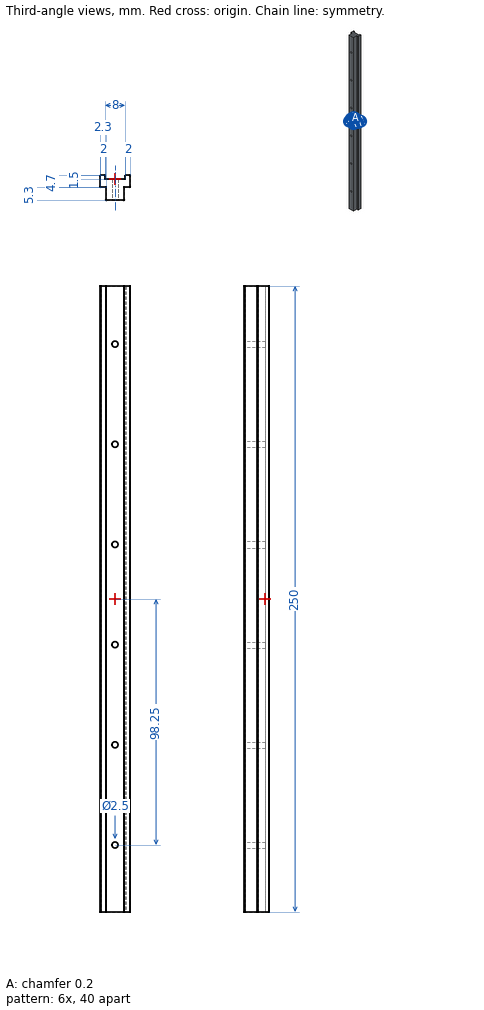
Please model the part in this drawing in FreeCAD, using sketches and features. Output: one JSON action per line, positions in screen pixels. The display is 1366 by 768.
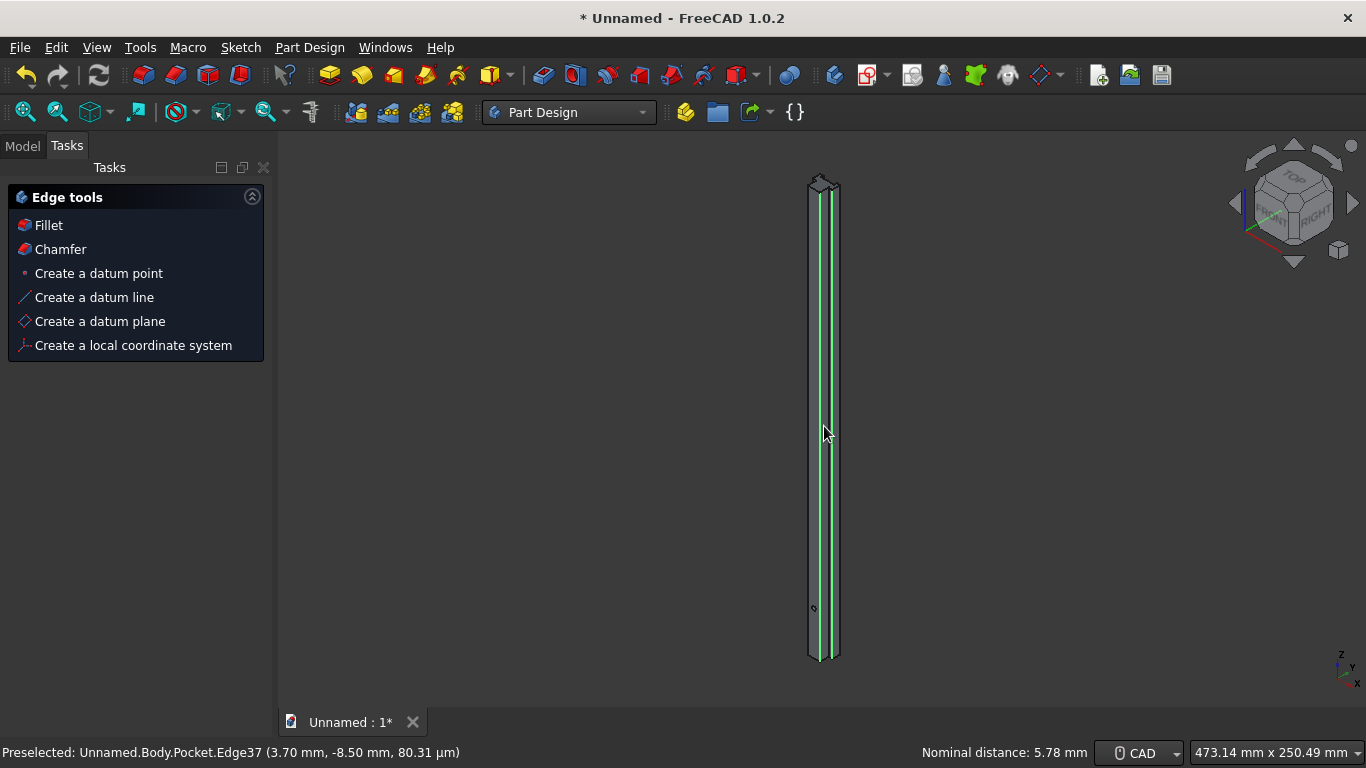
{"action": "key", "text": "2"}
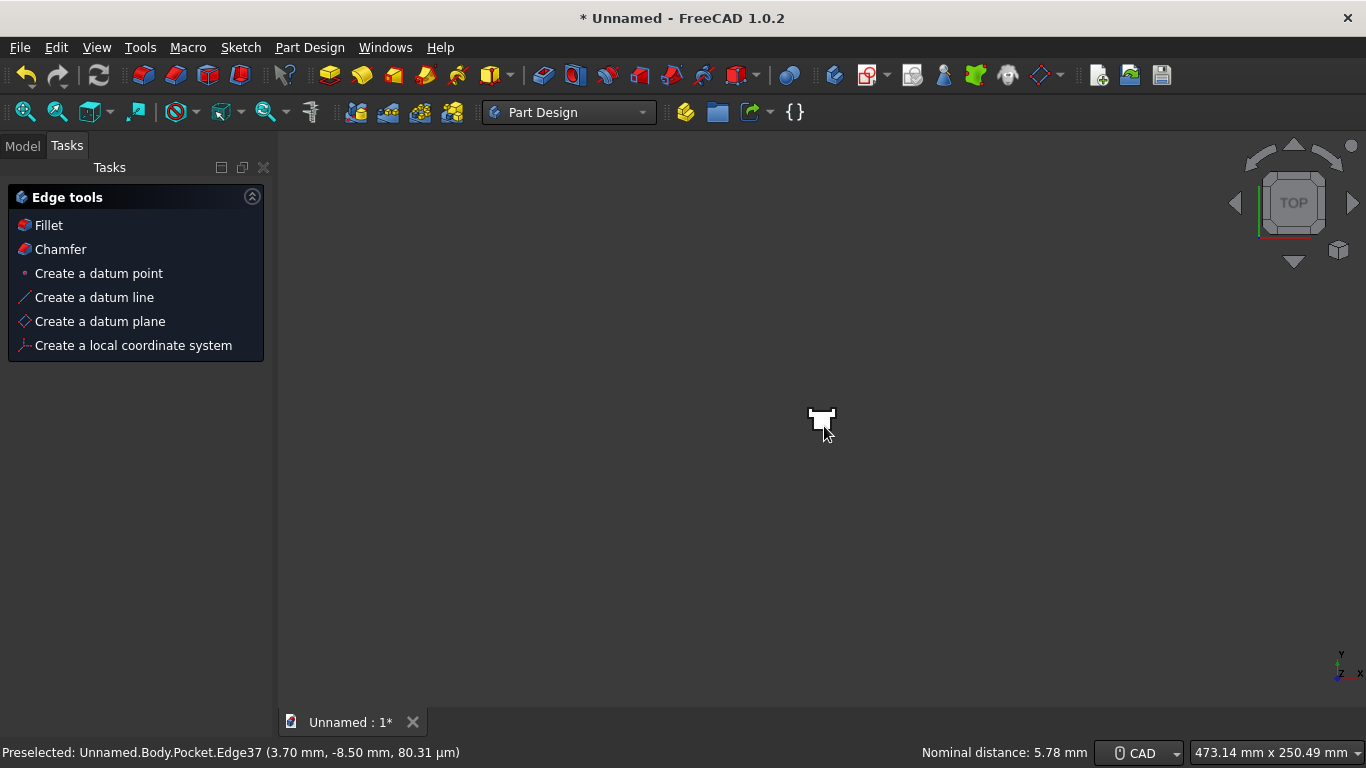
{"action": "left_click", "coordinate": [26, 112]}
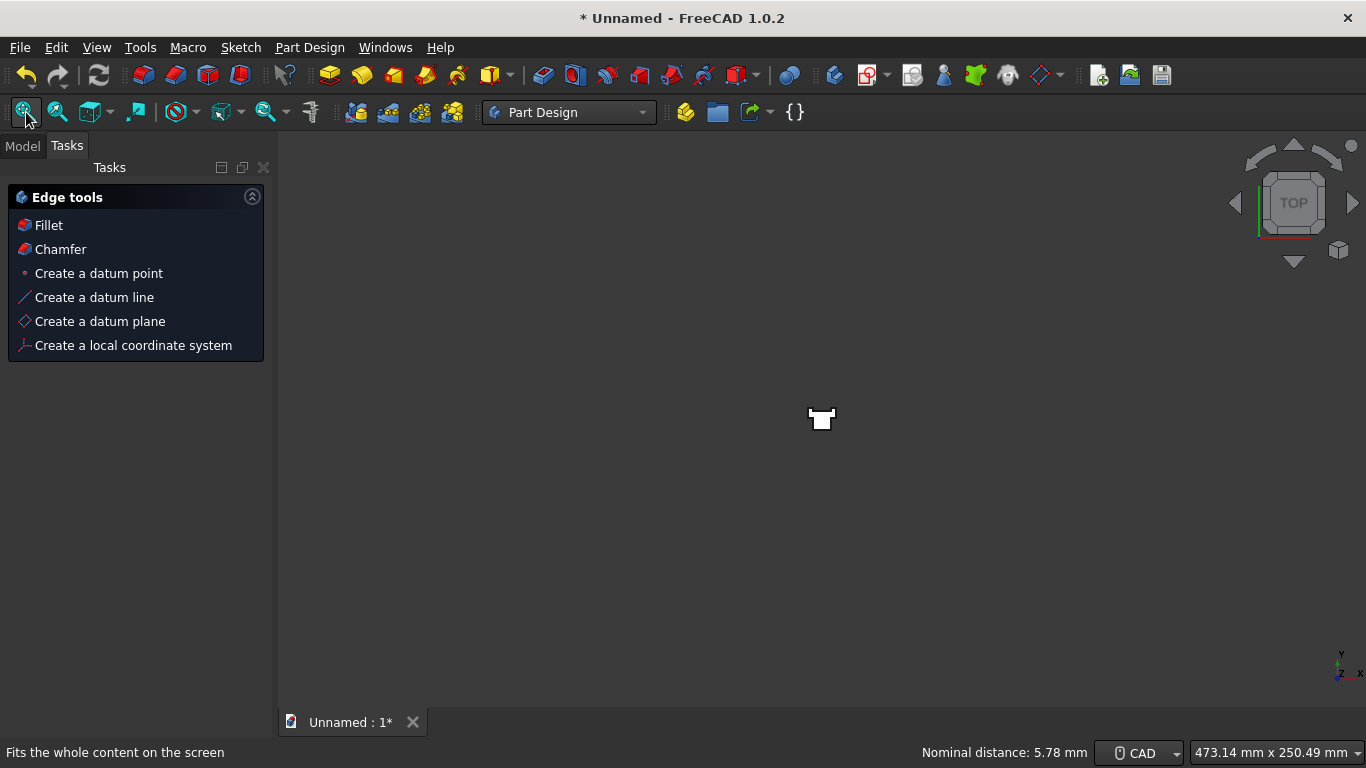
{"action": "key", "text": "1"}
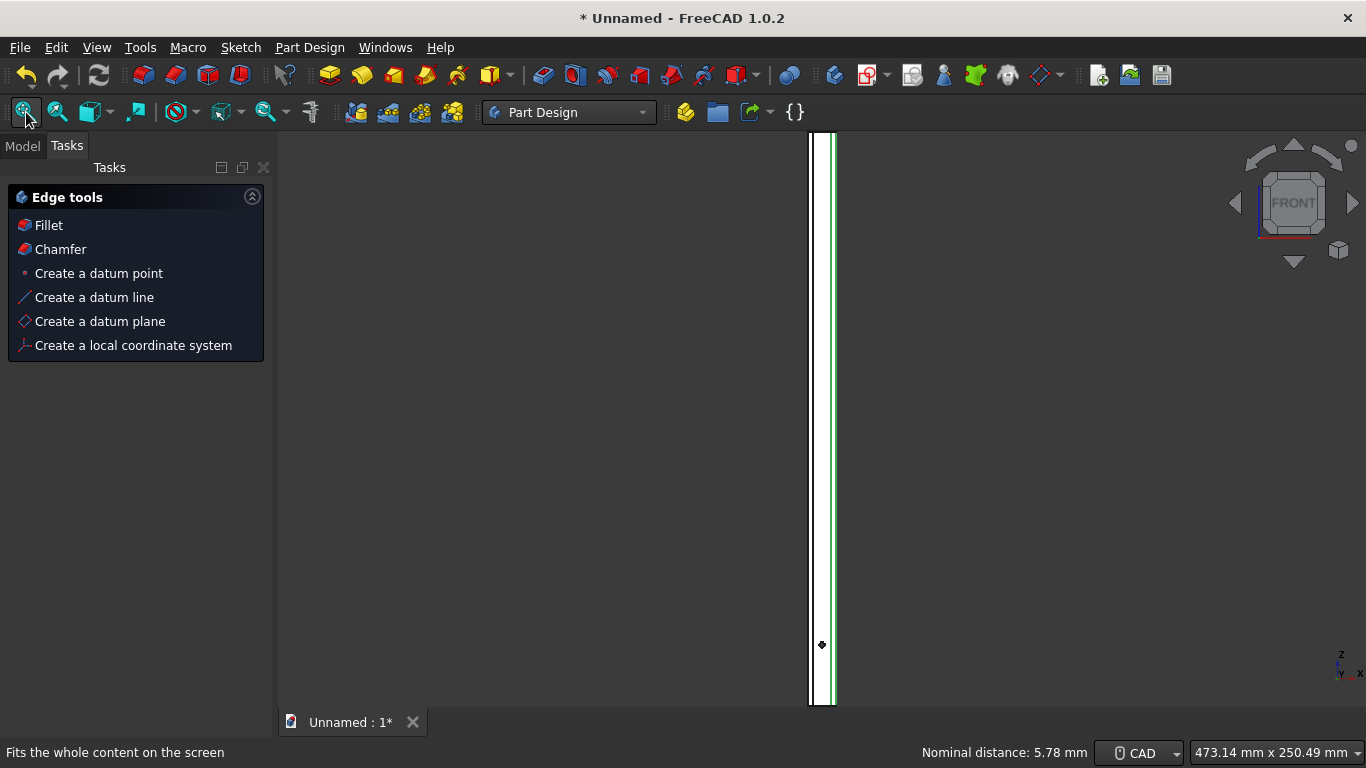
{"action": "left_click", "coordinate": [813, 418], "text": "ctrl"}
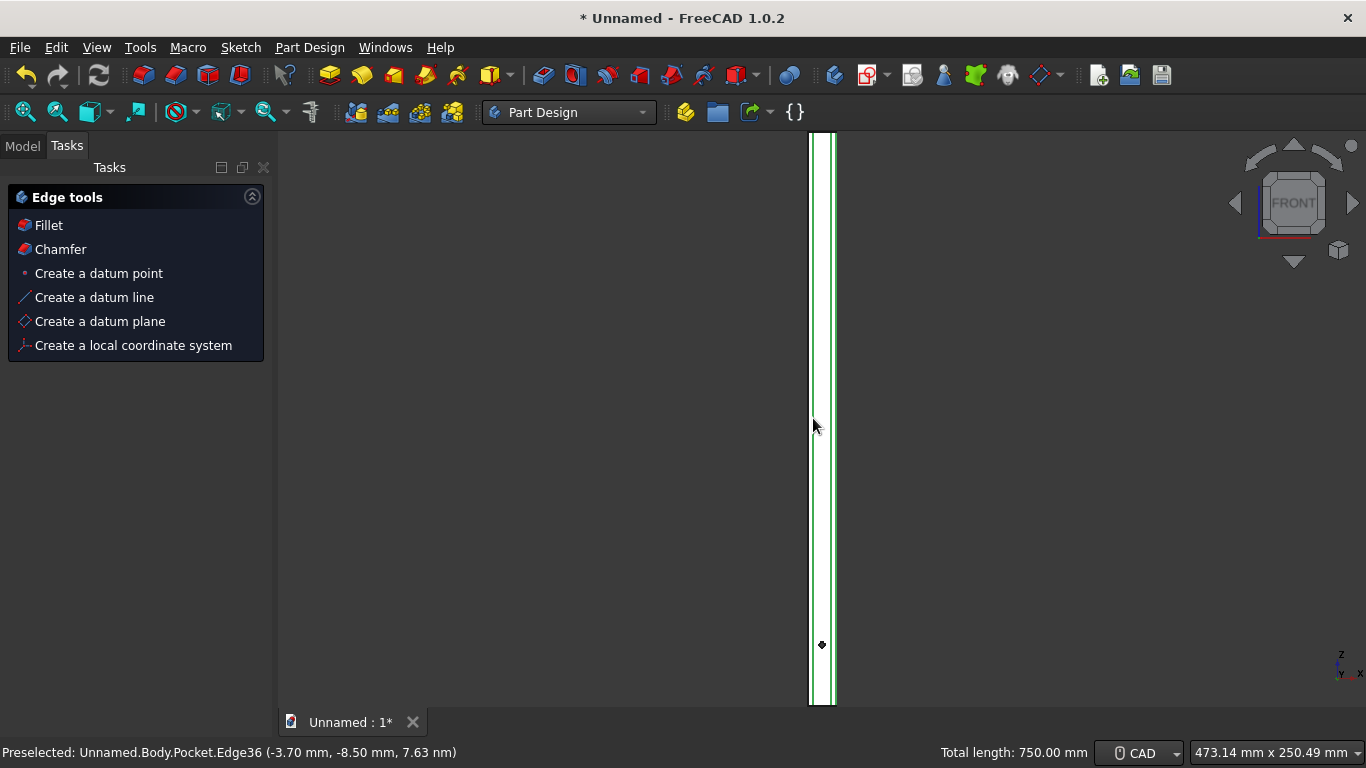
{"action": "key", "text": "3"}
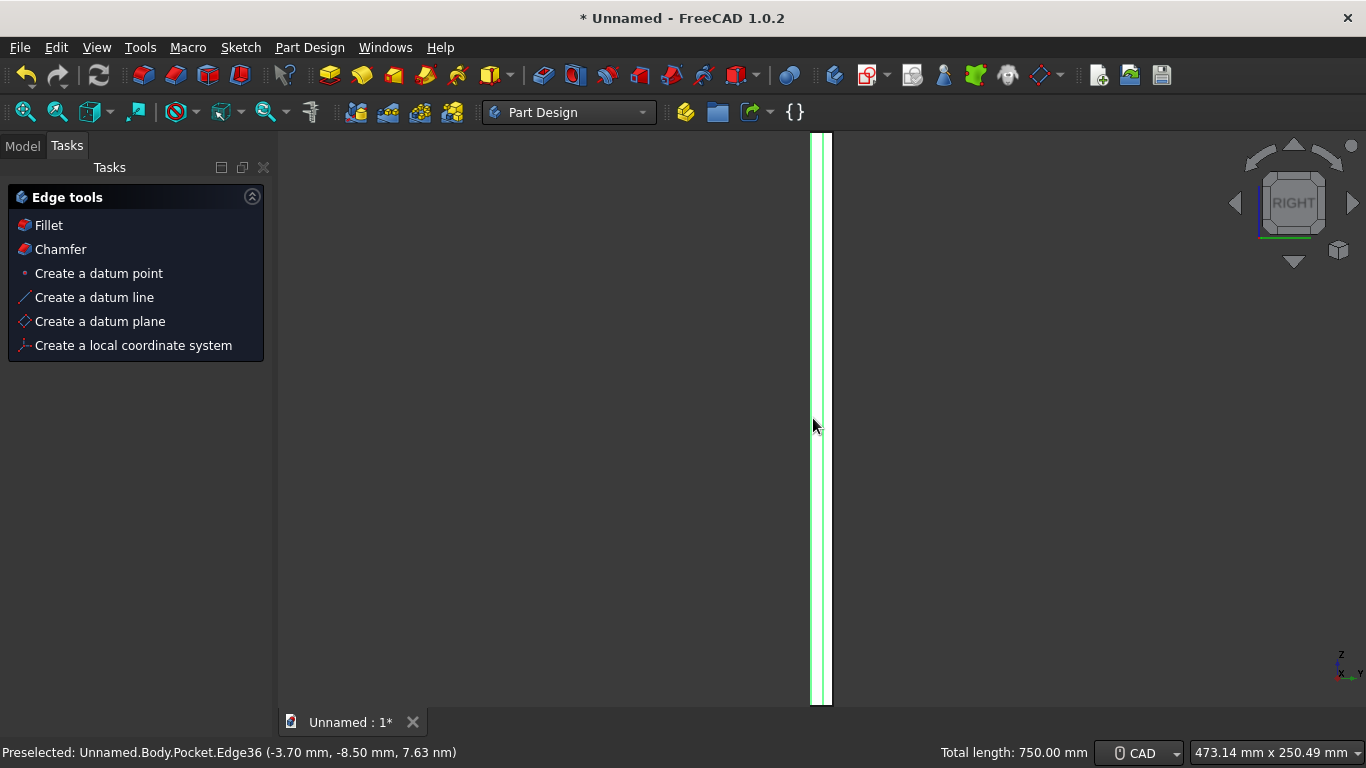
{"action": "left_click", "coordinate": [833, 418], "text": "ctrl"}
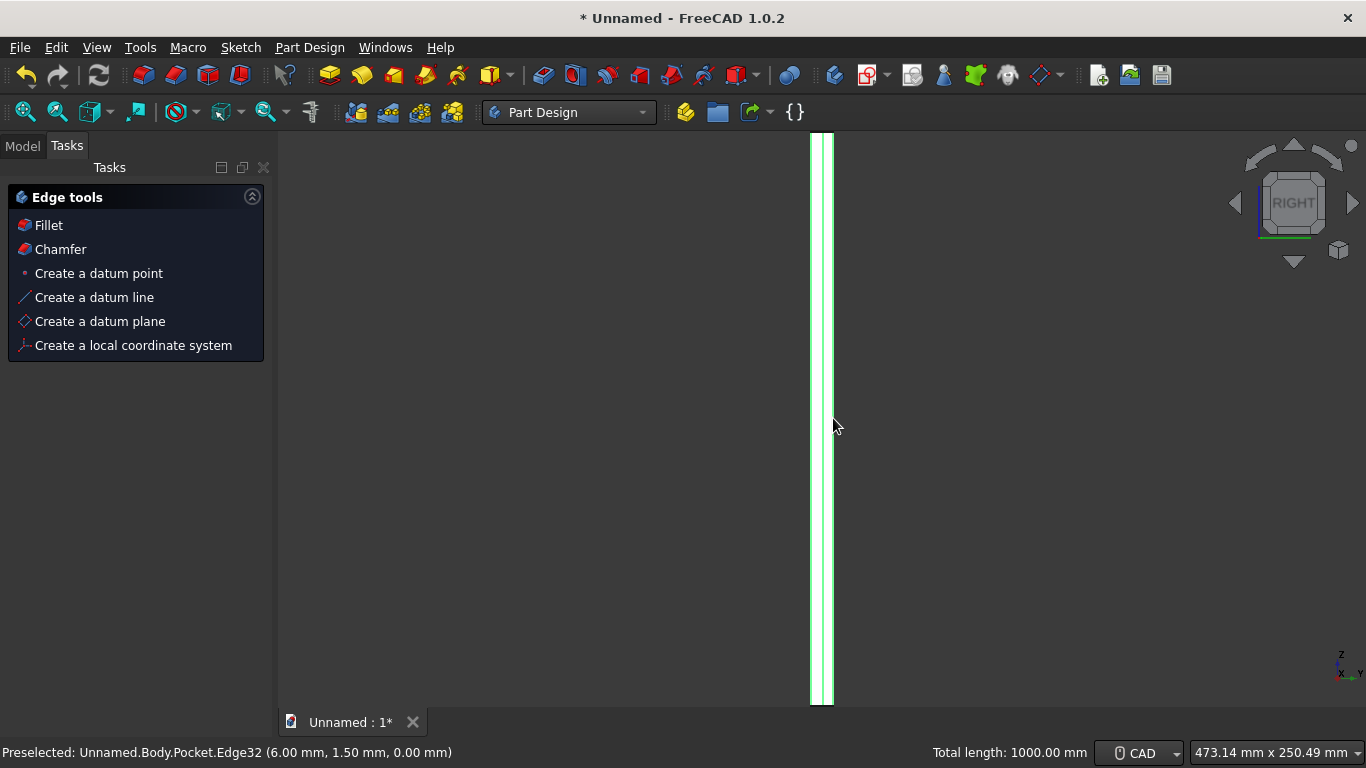
{"action": "key", "text": "5"}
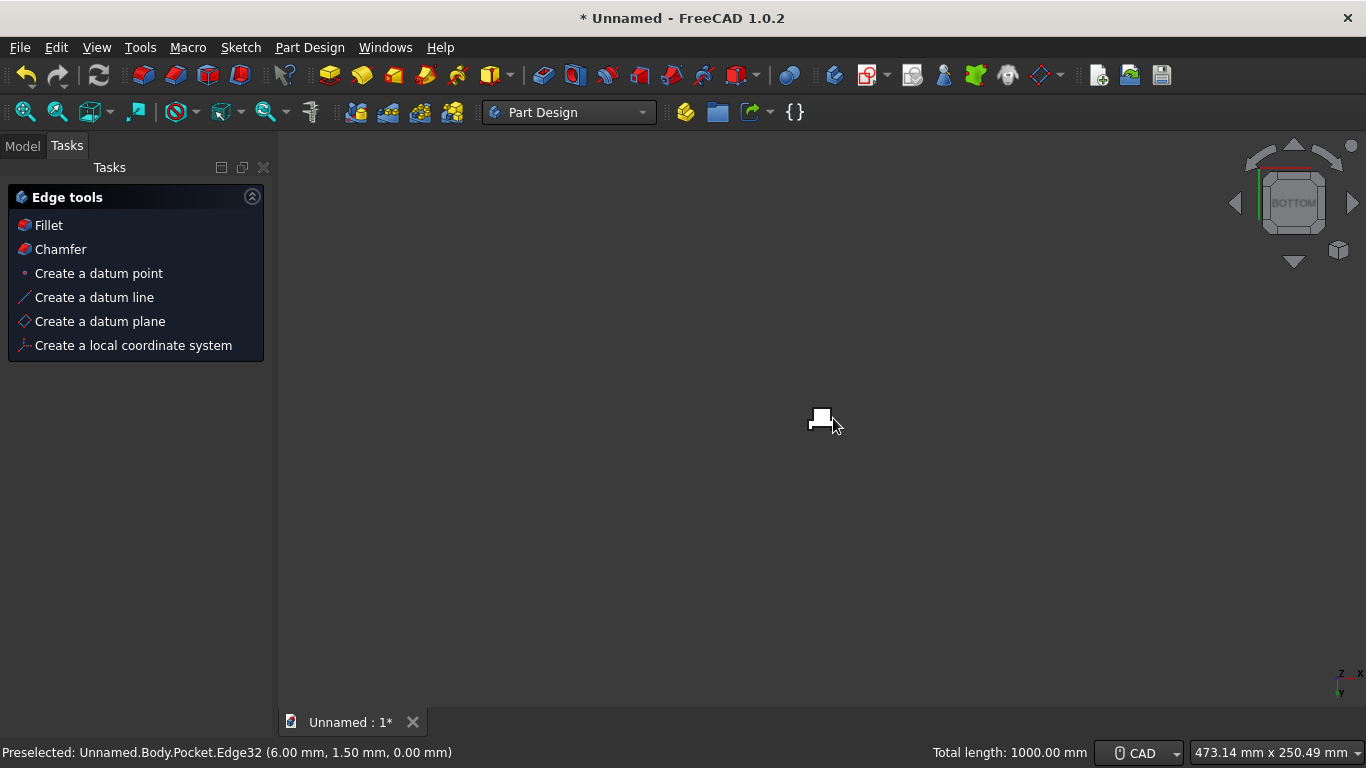
{"action": "left_click", "coordinate": [26, 112]}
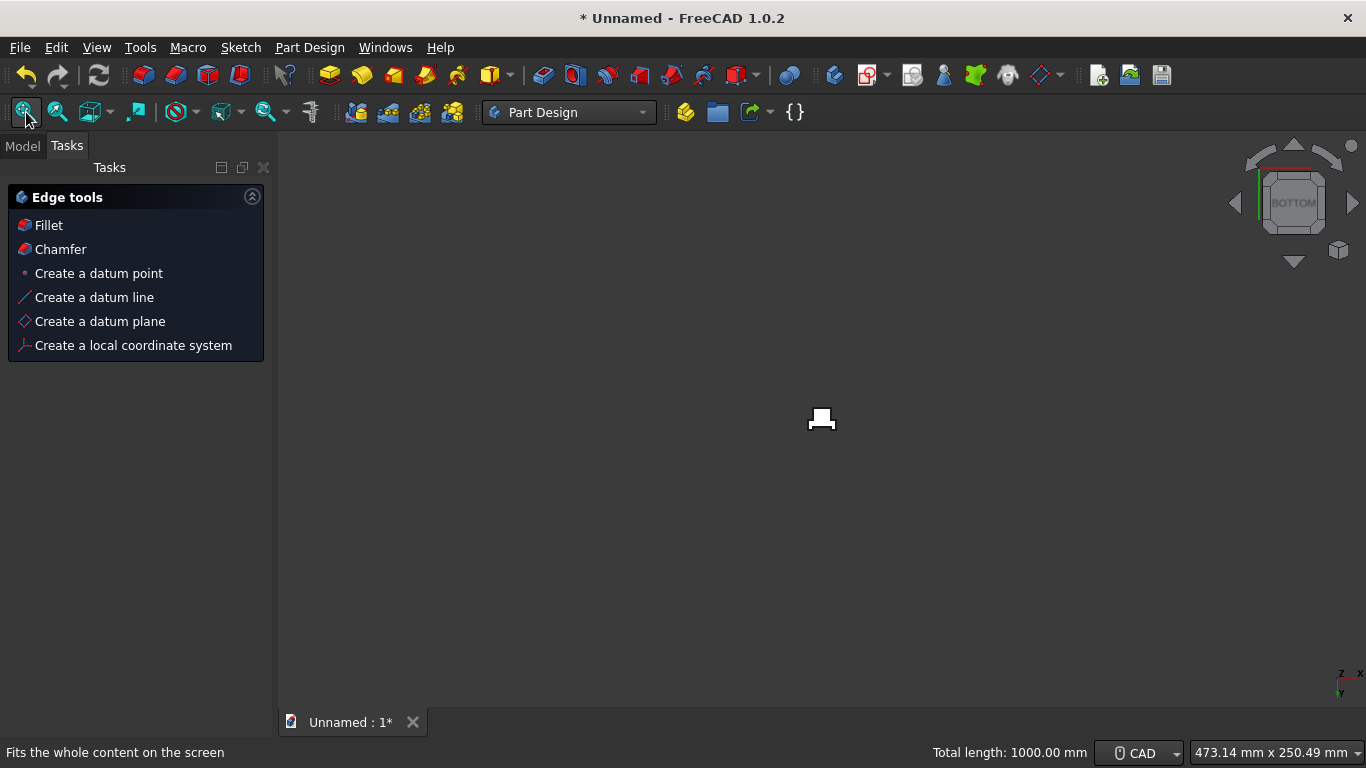
{"action": "key", "text": "4"}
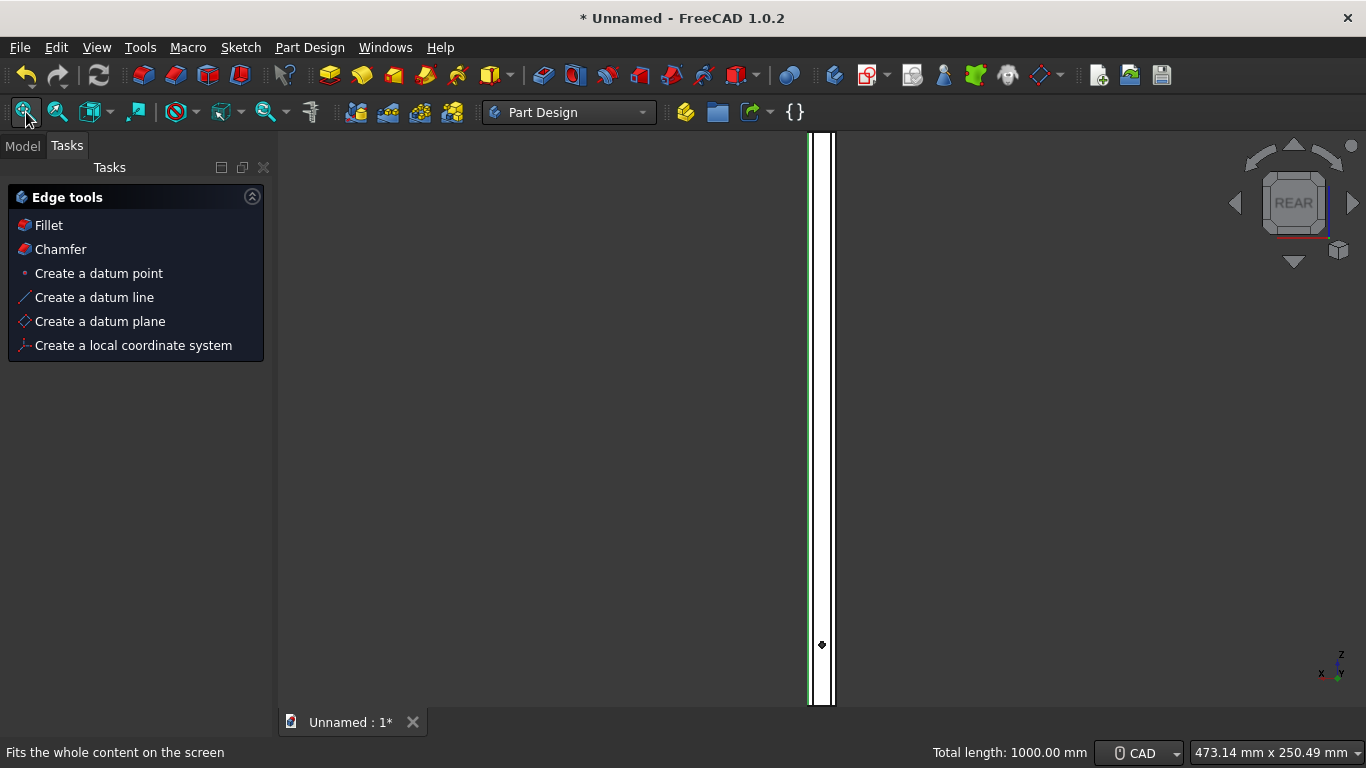
{"action": "left_click", "coordinate": [813, 418], "text": "ctrl"}